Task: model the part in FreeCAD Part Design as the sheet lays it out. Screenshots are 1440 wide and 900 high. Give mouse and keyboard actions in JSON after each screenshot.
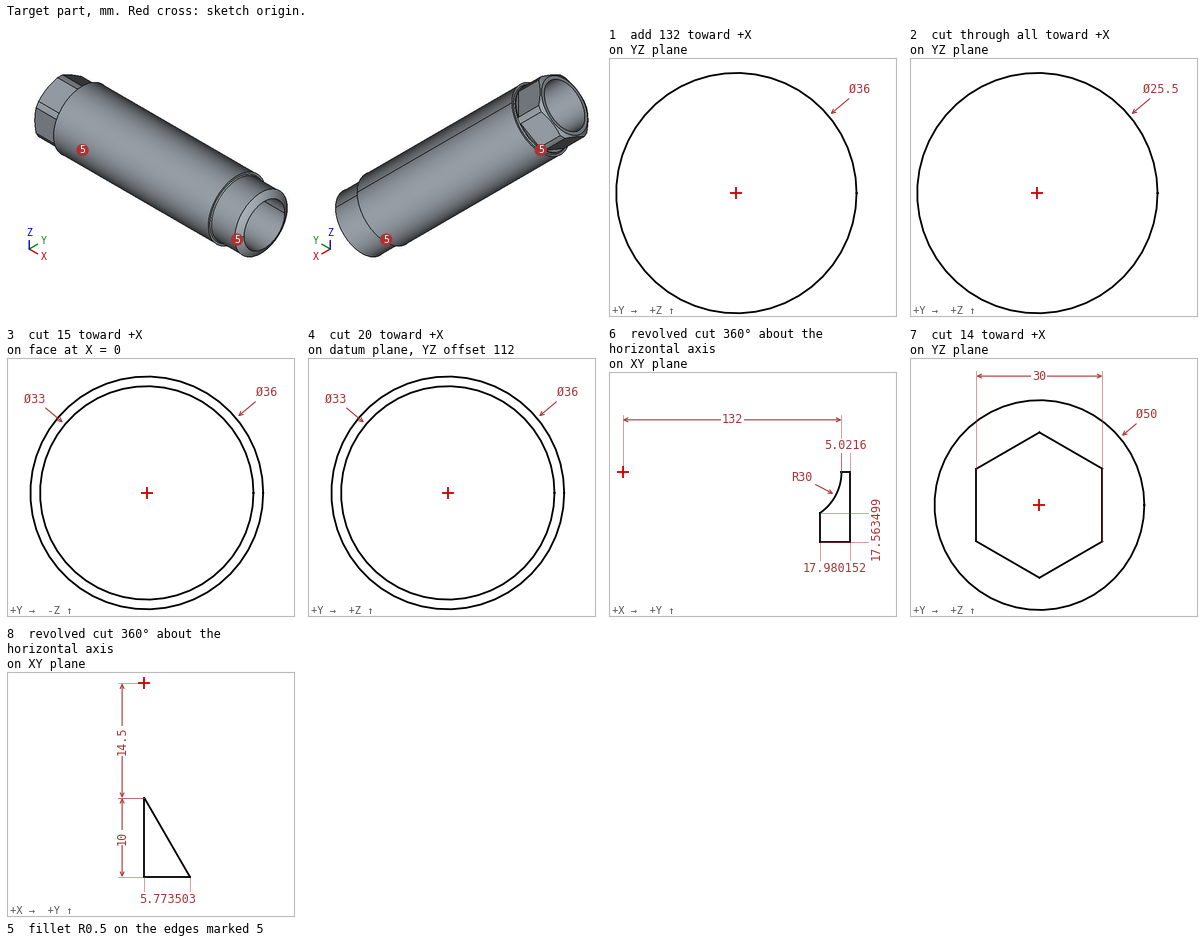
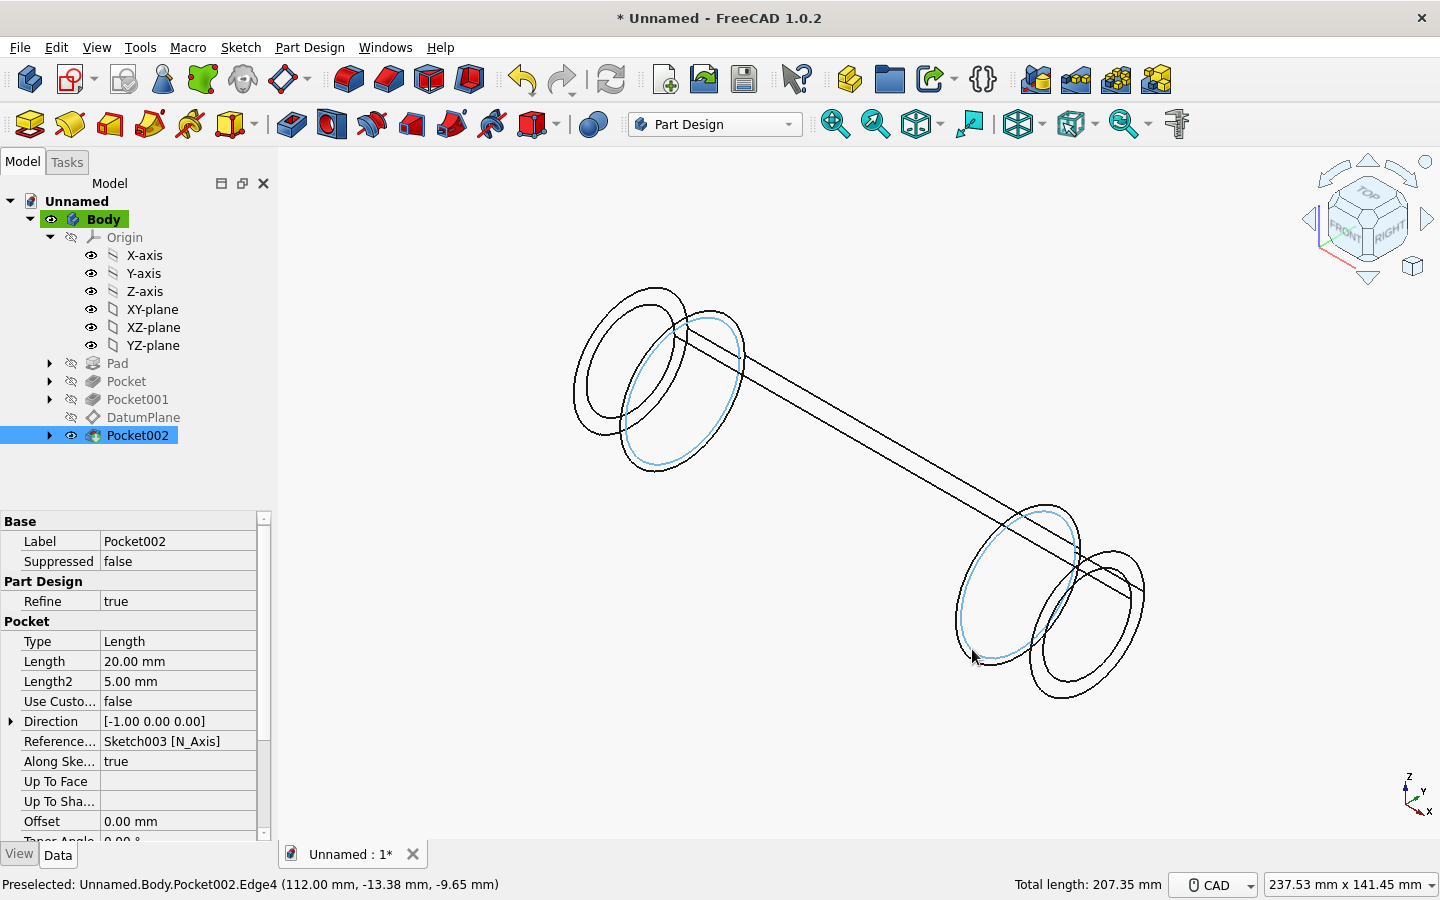
{"action": "key", "text": "v 1"}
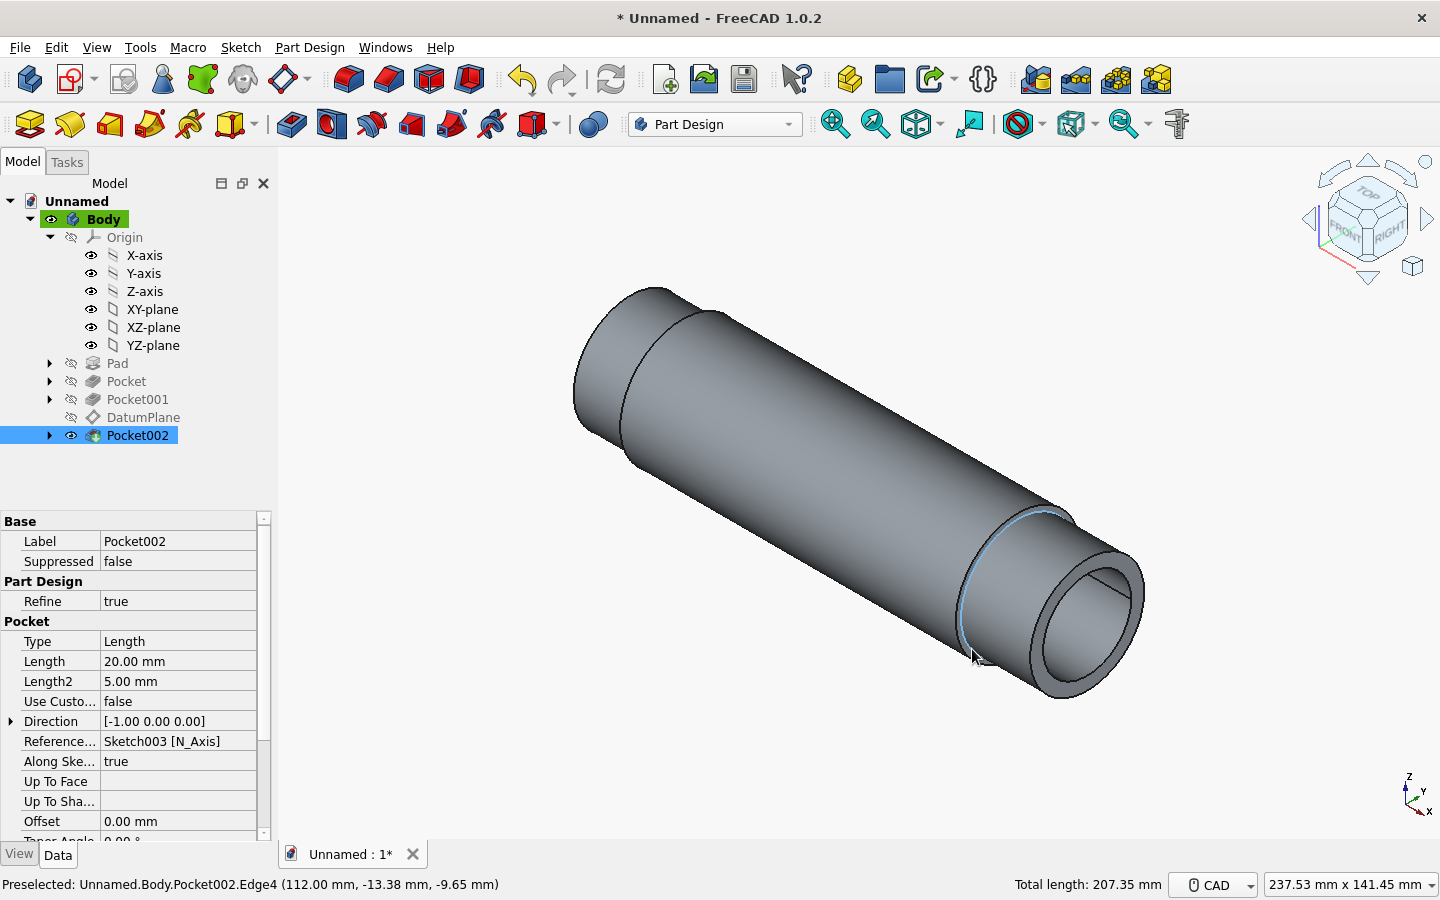
{"action": "left_click", "coordinate": [350, 80]}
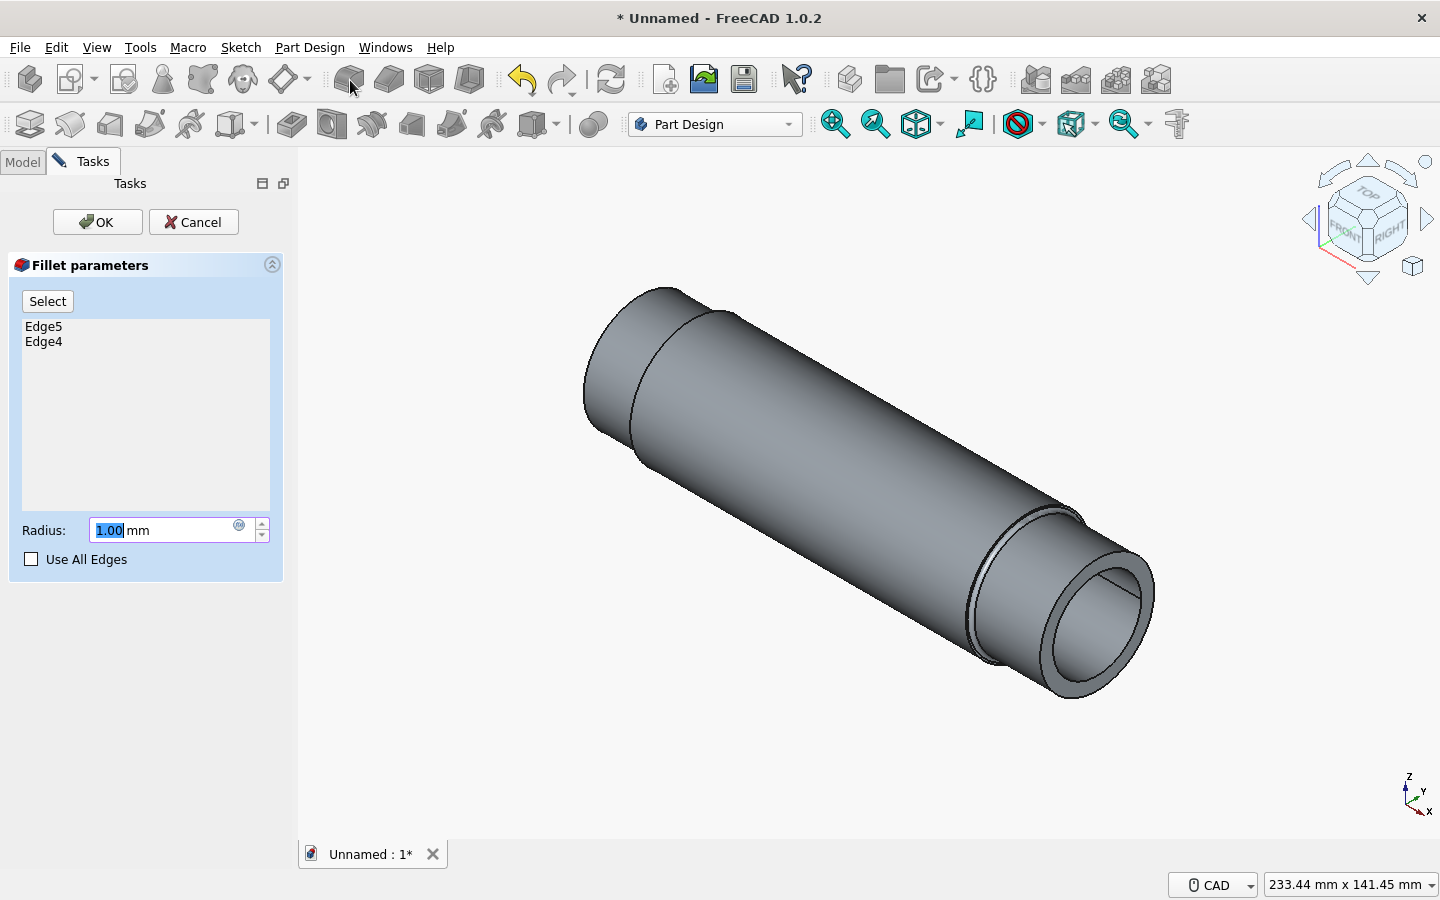
{"action": "type", "text": "0.5"}
{"action": "key", "text": "Tab"}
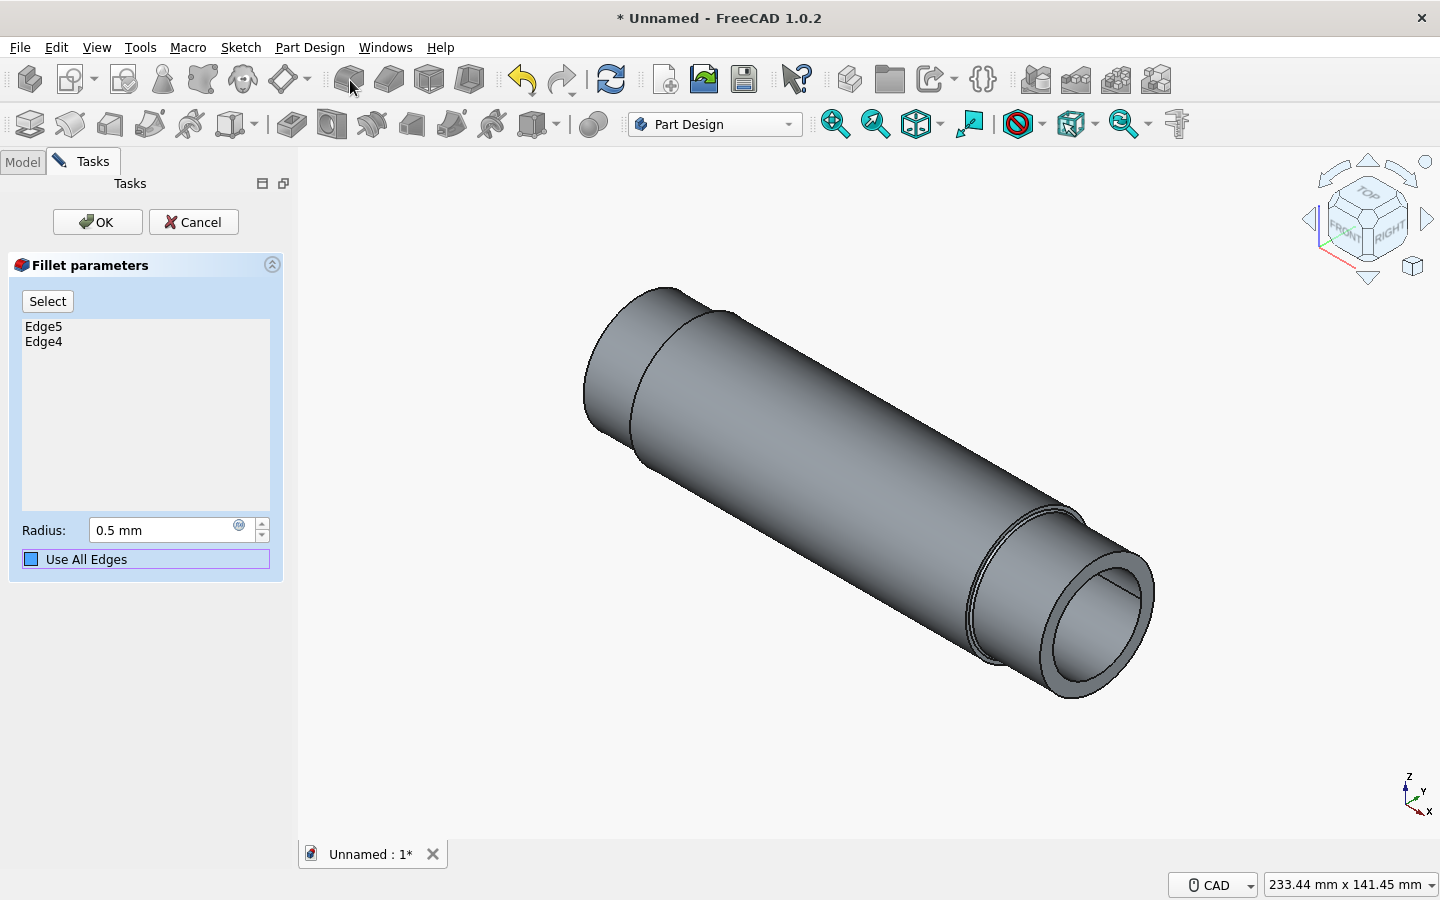
{"action": "left_click", "coordinate": [98, 222]}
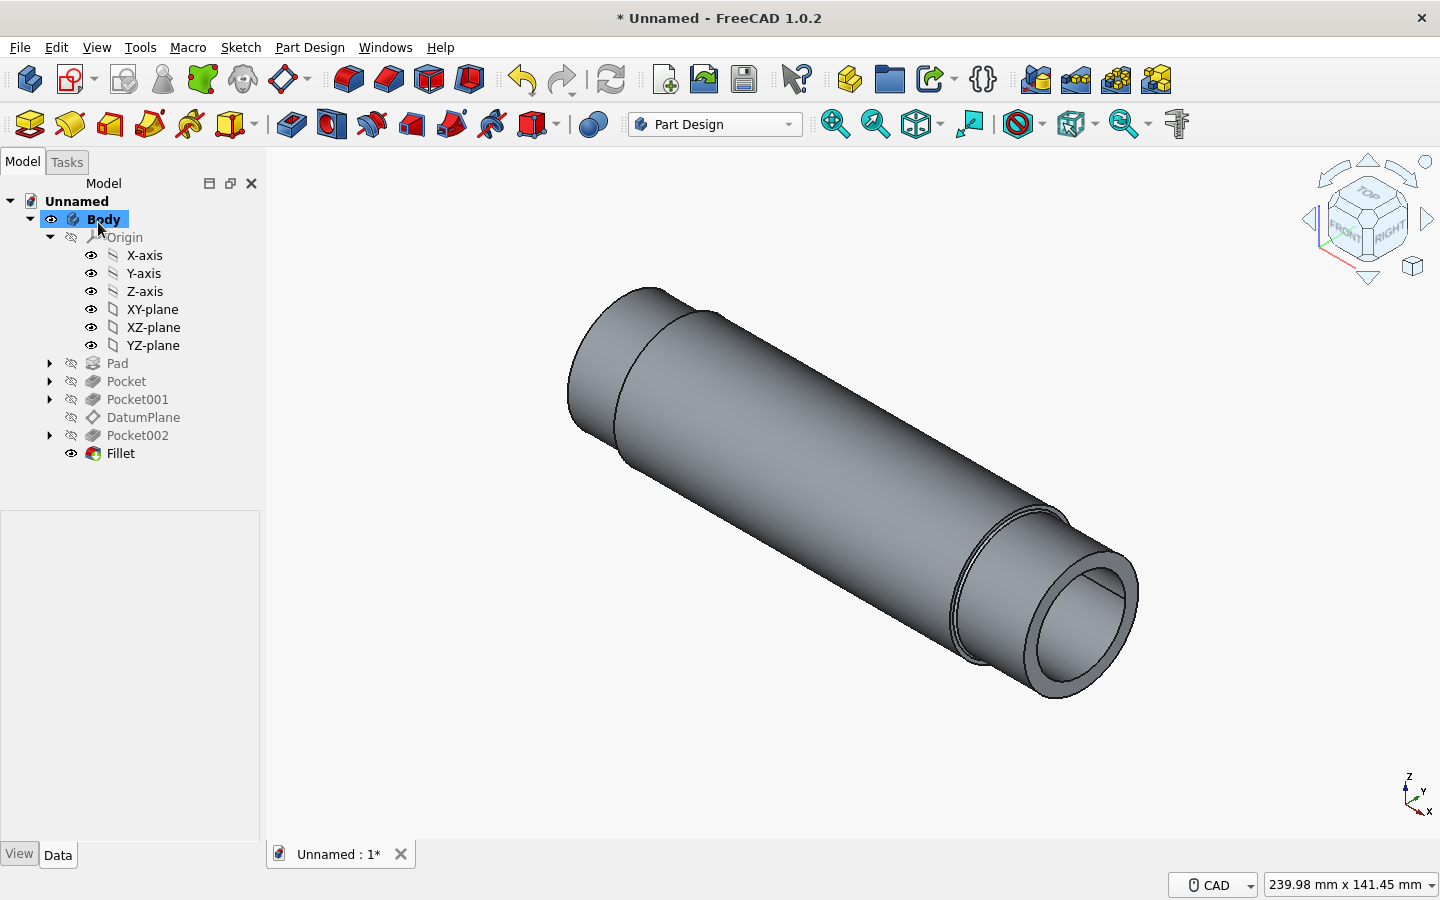
{"action": "left_click", "coordinate": [70, 80]}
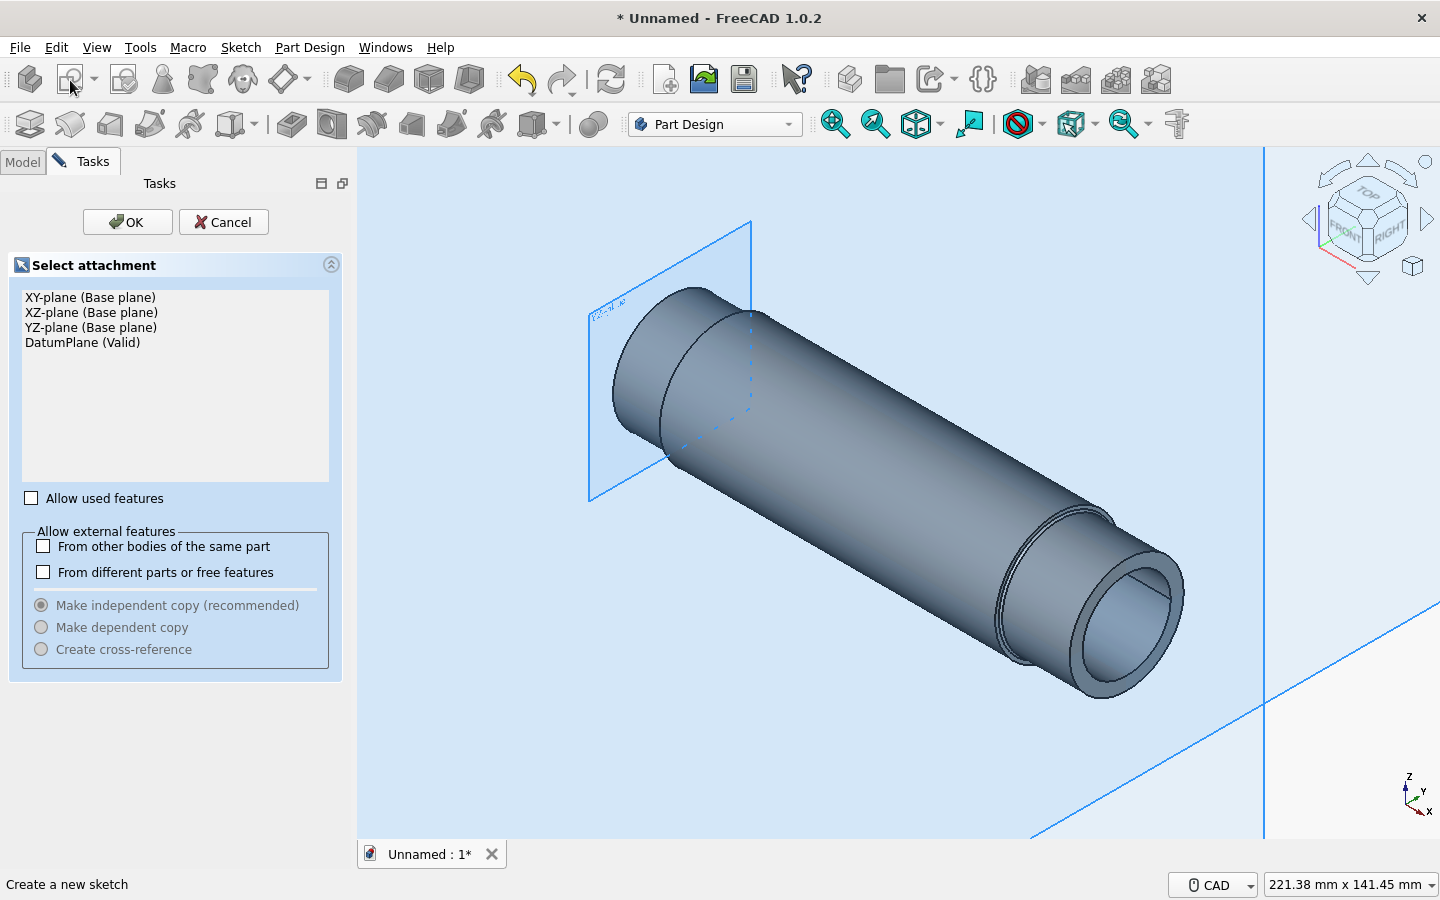
{"action": "left_click", "coordinate": [82, 298]}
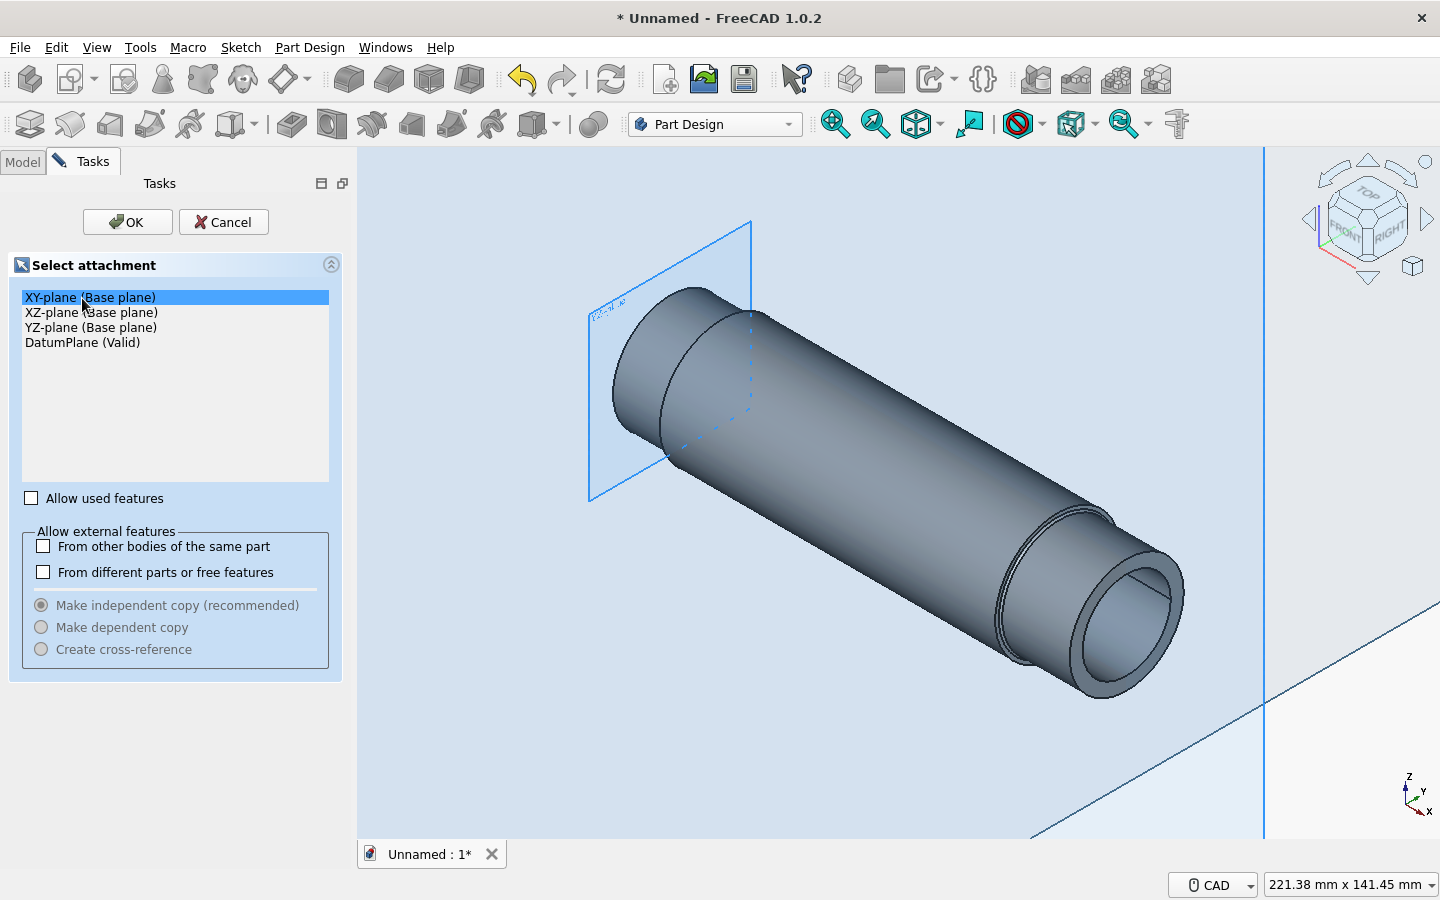
{"action": "left_click", "coordinate": [128, 222]}